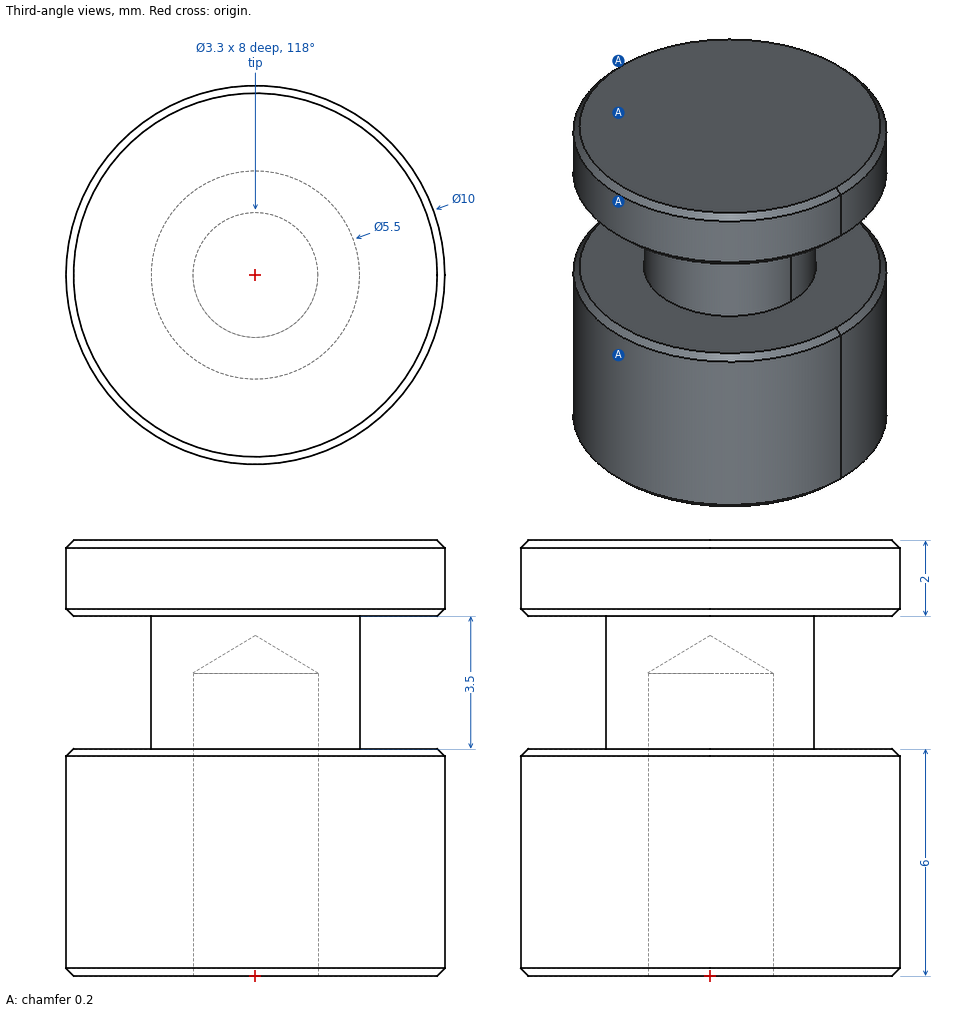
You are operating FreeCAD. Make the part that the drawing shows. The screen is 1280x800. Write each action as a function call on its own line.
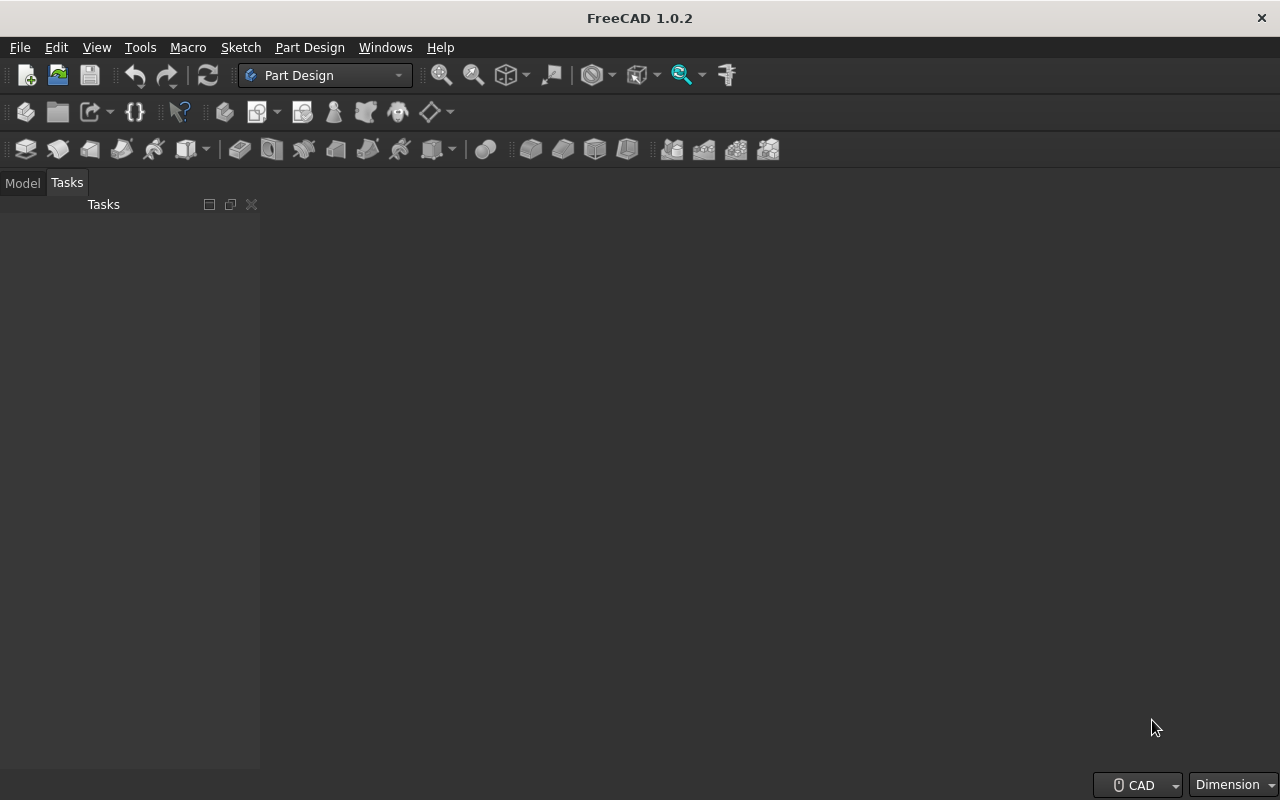
key(ctrl+n)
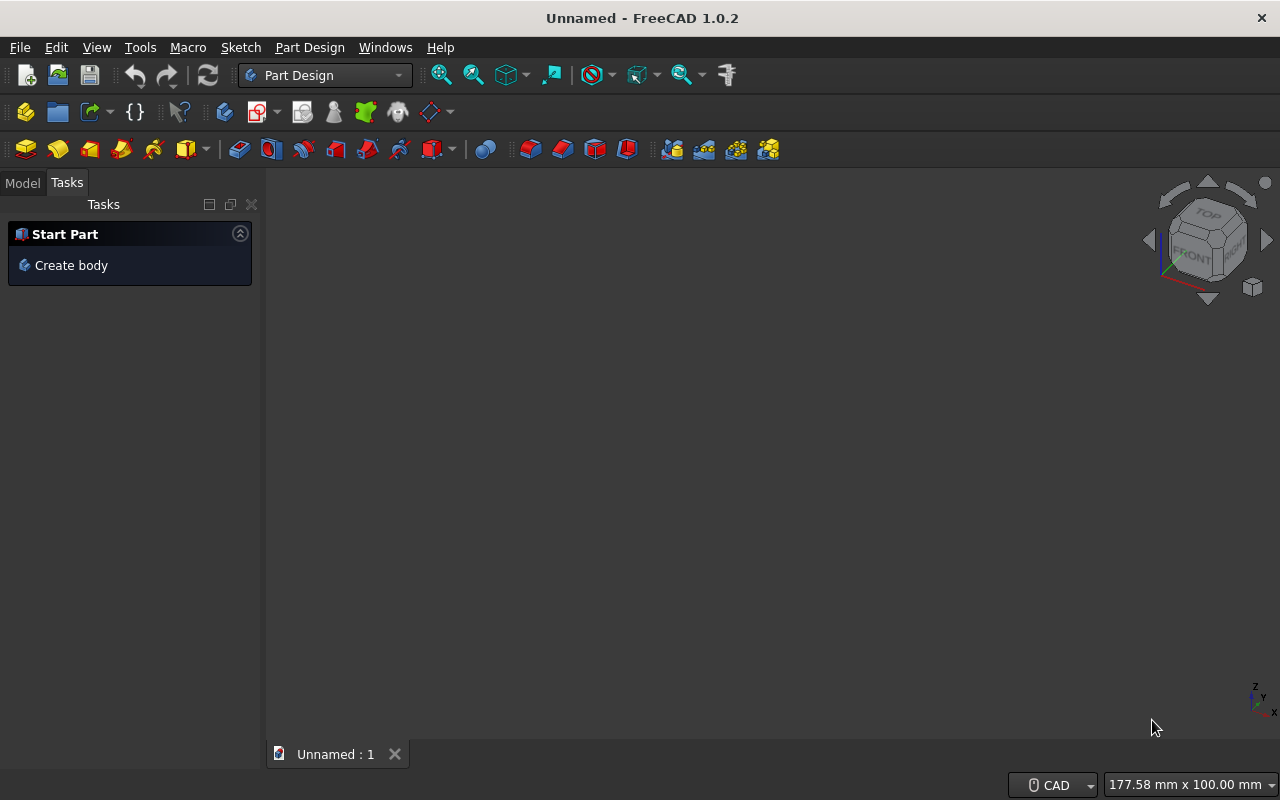
click(258, 112)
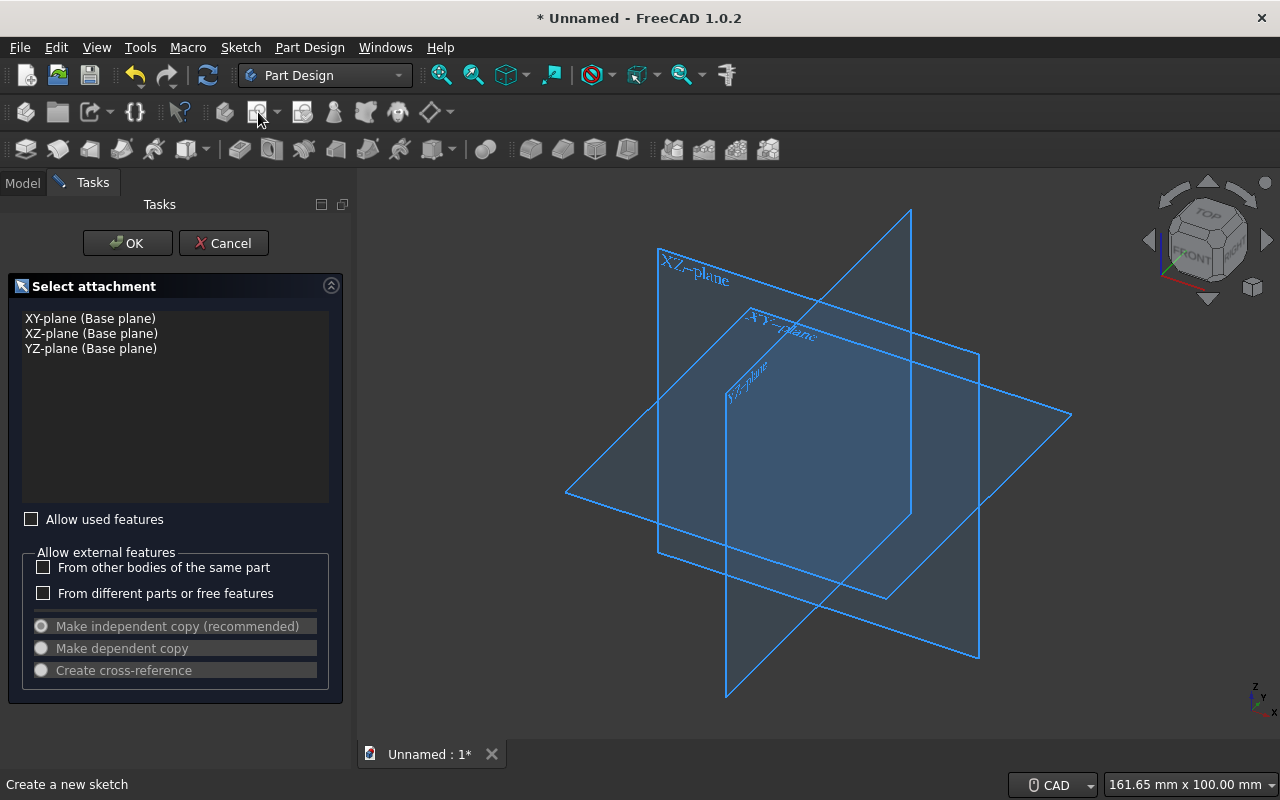
click(82, 318)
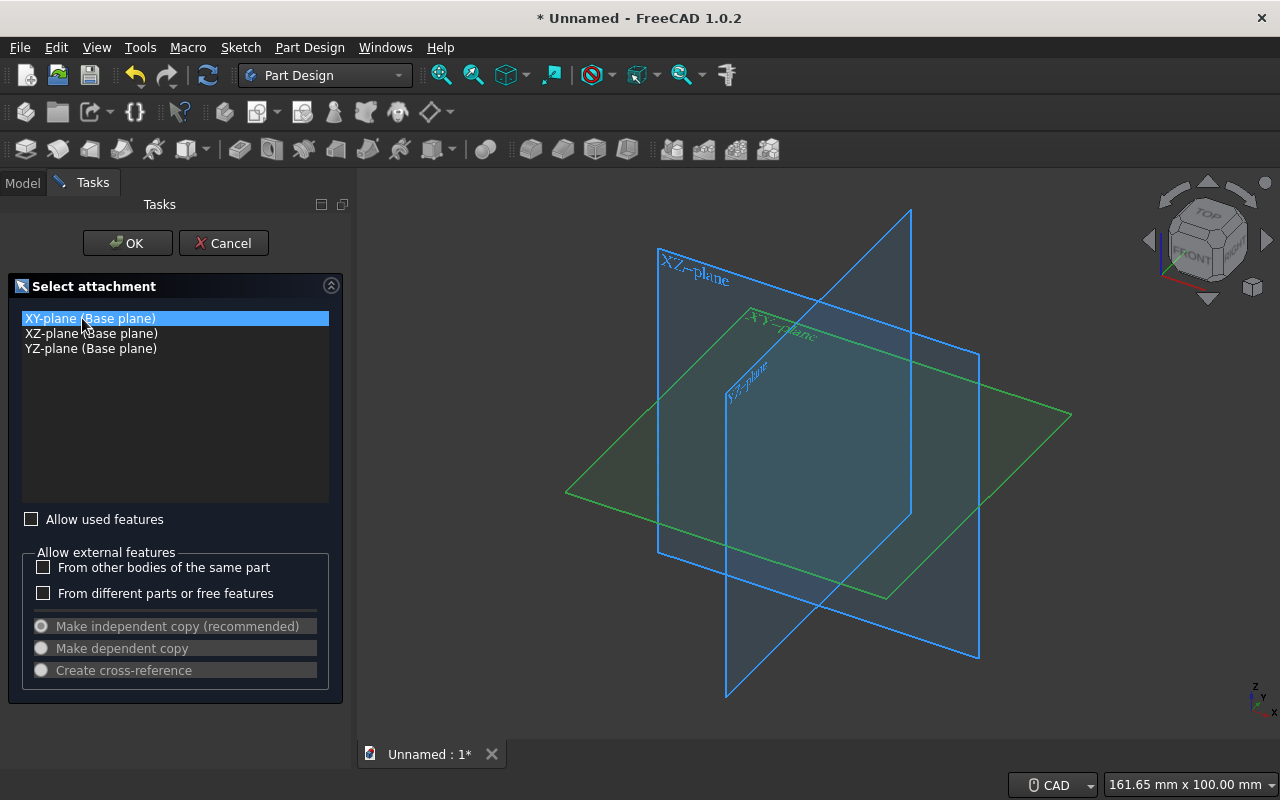
click(128, 243)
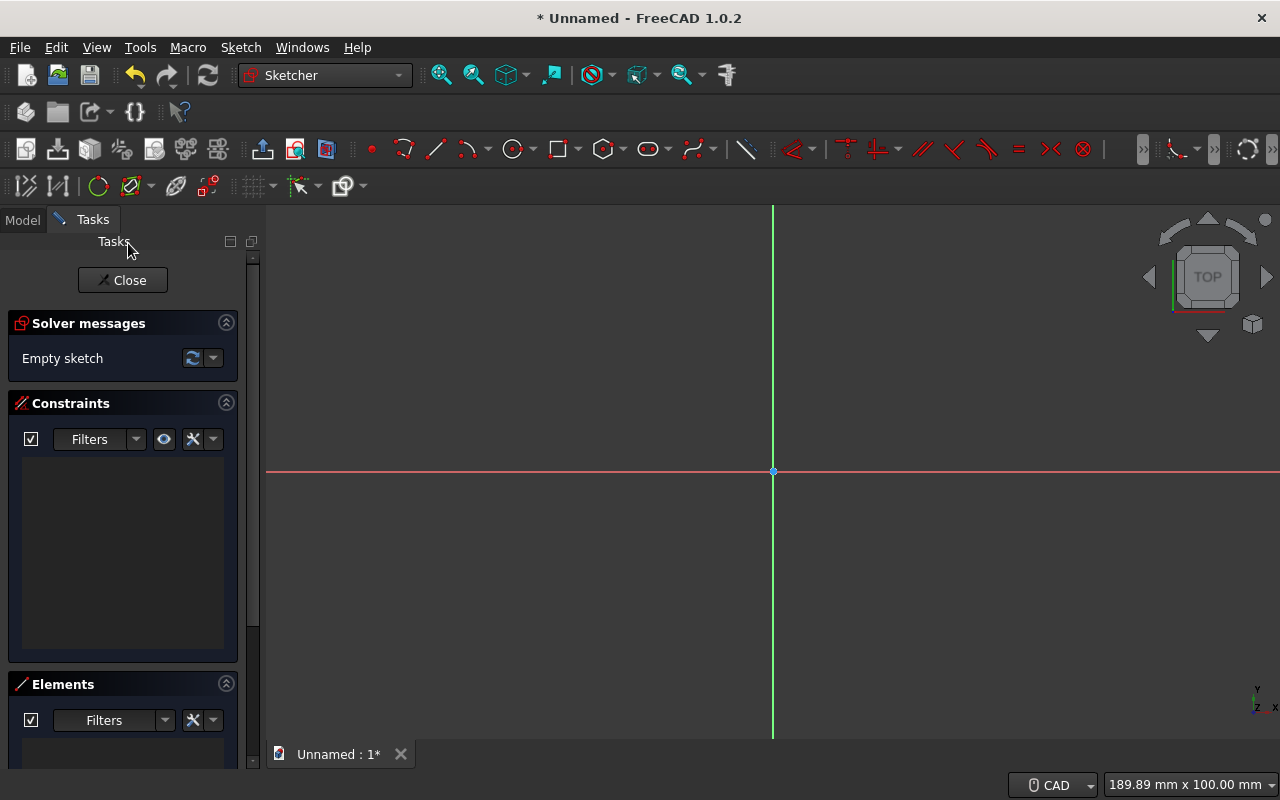
scroll(787, 472, up, 9)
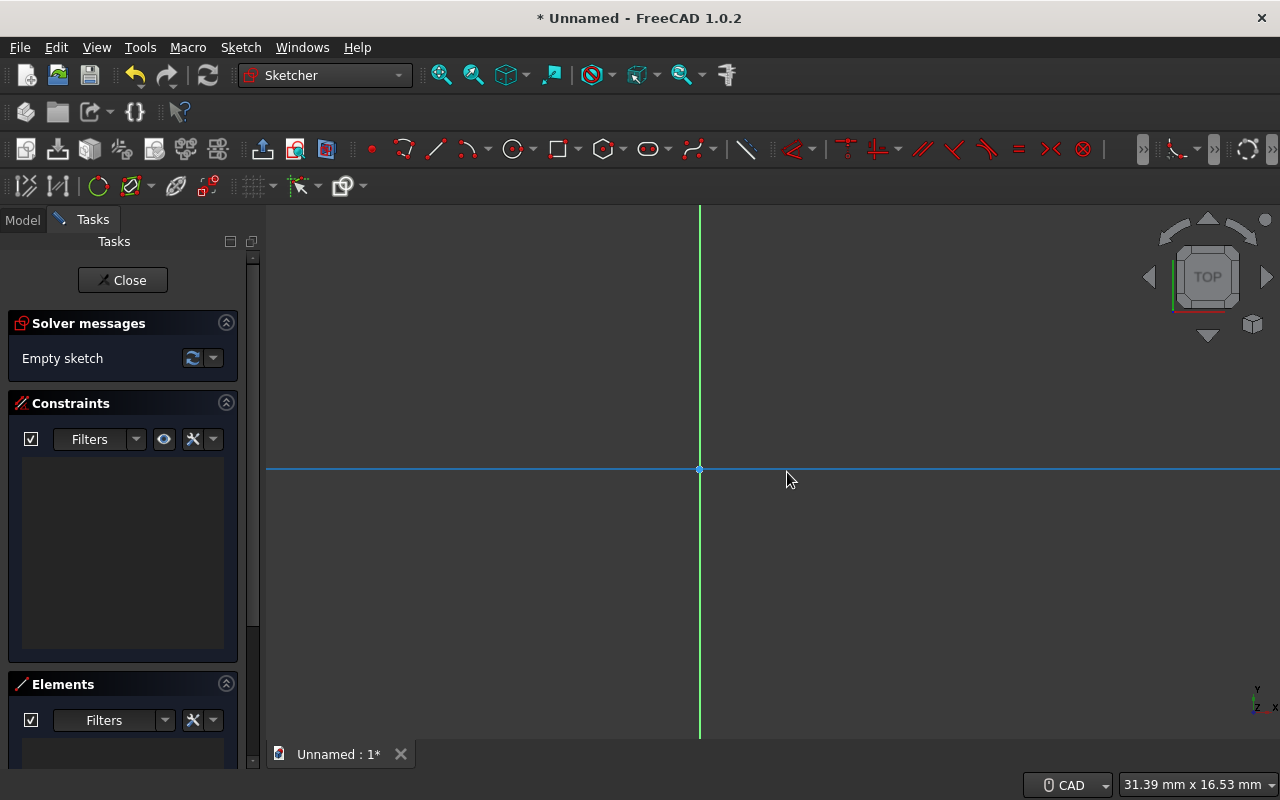
click(514, 150)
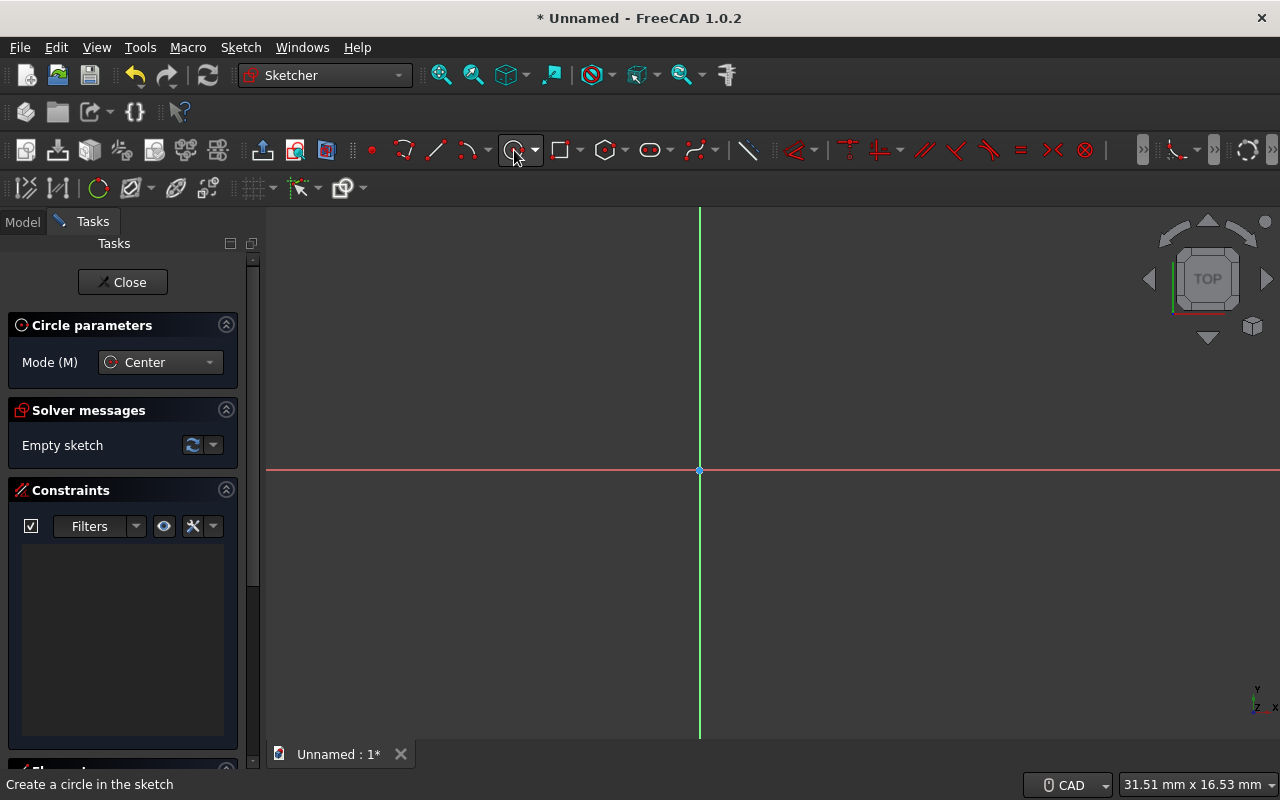
click(700, 470)
move(814, 357)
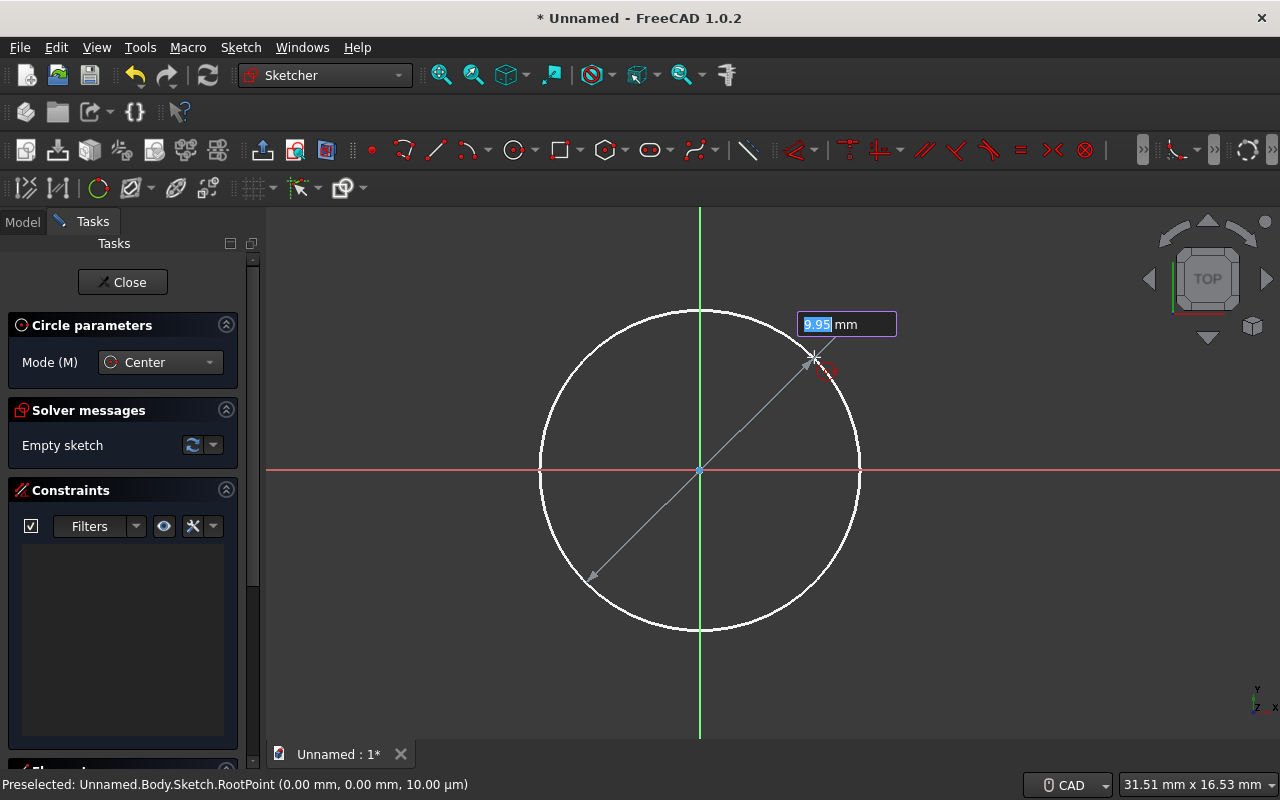
text(10)
key(Return)
key(Escape)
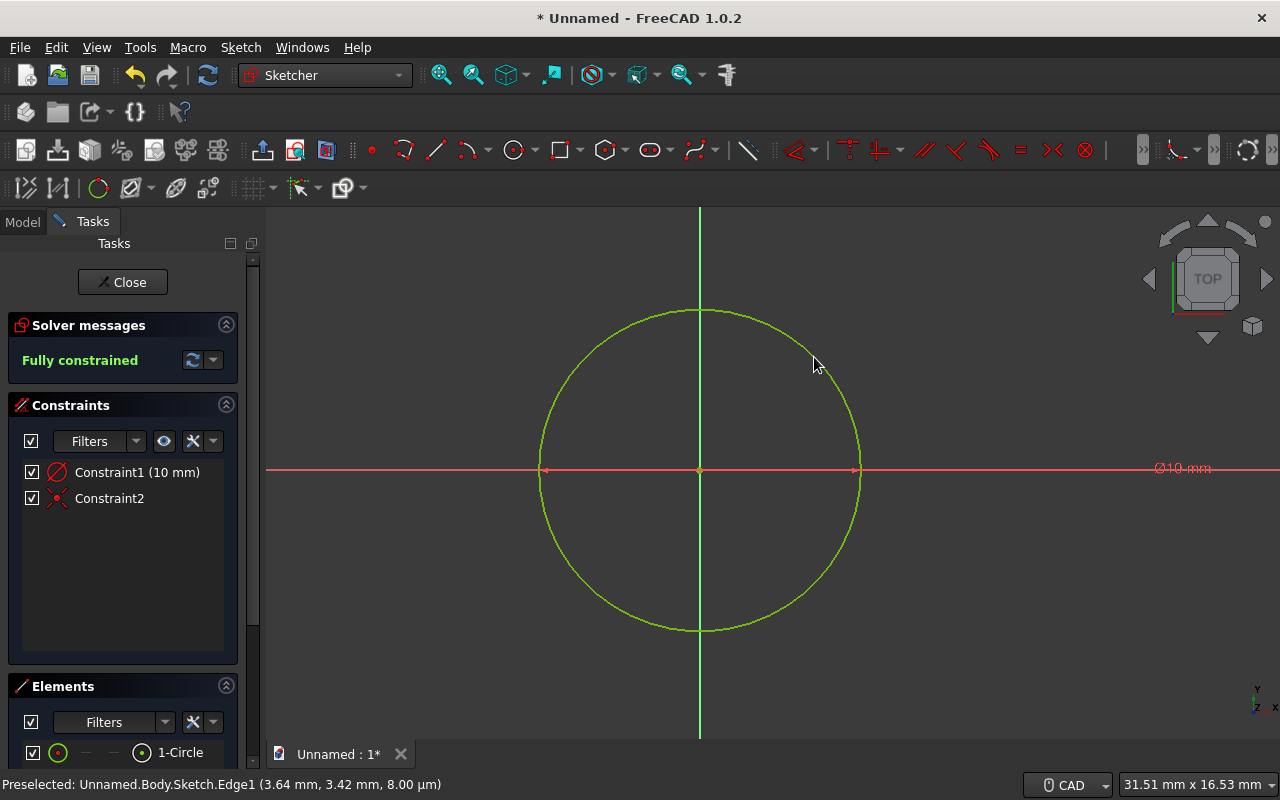
click(123, 282)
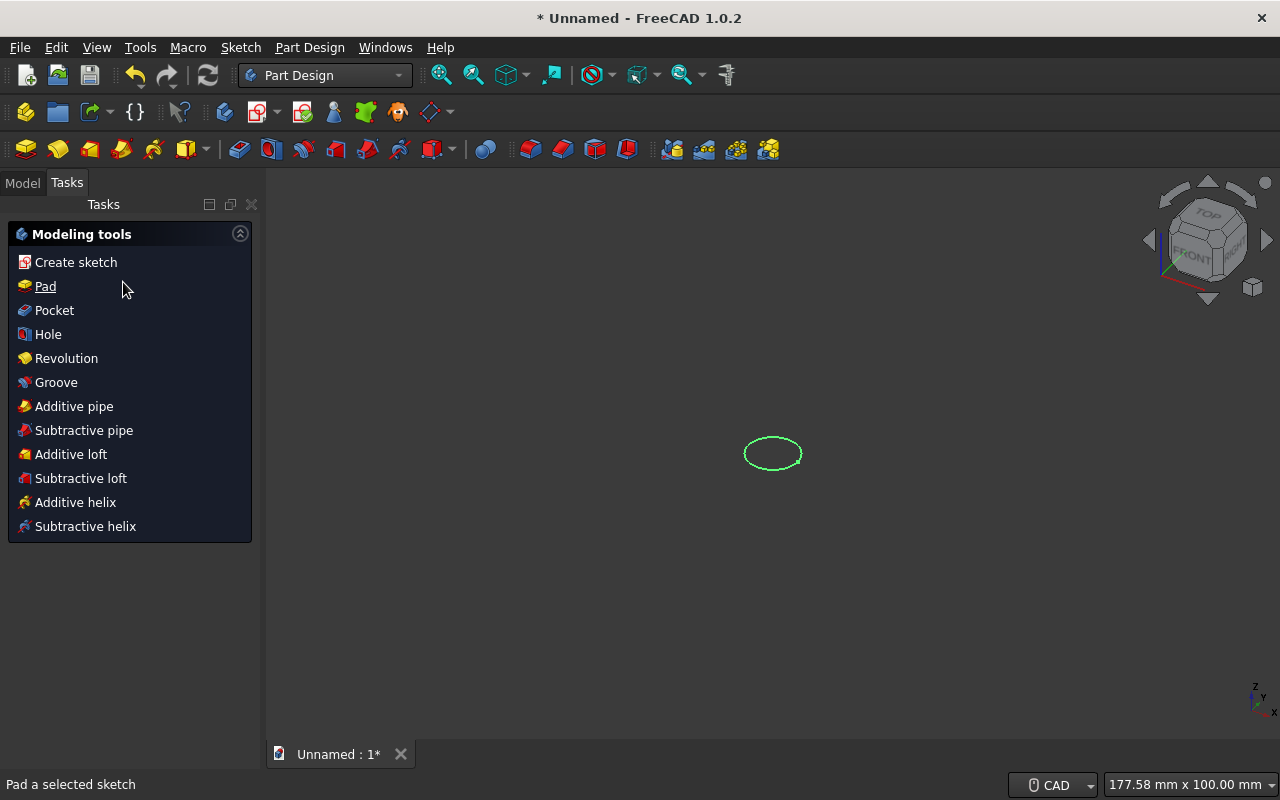
click(26, 150)